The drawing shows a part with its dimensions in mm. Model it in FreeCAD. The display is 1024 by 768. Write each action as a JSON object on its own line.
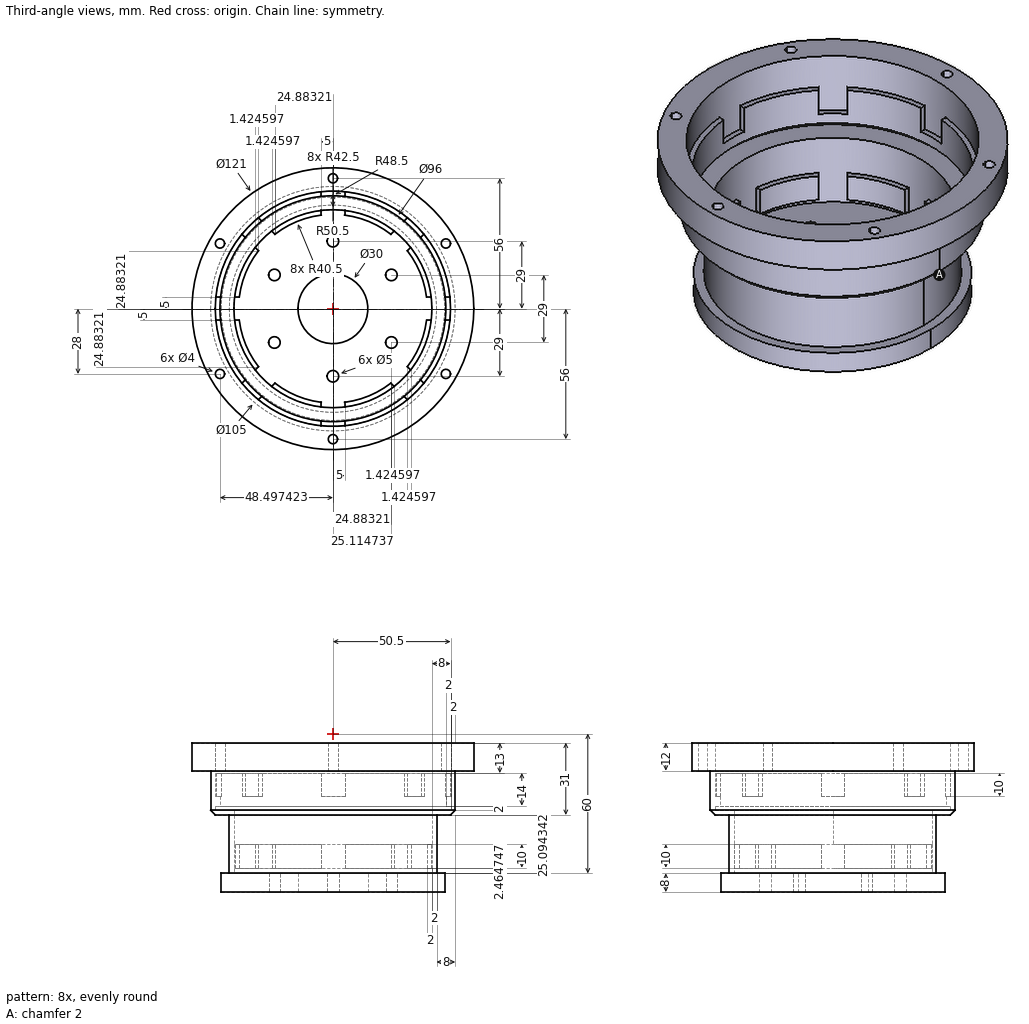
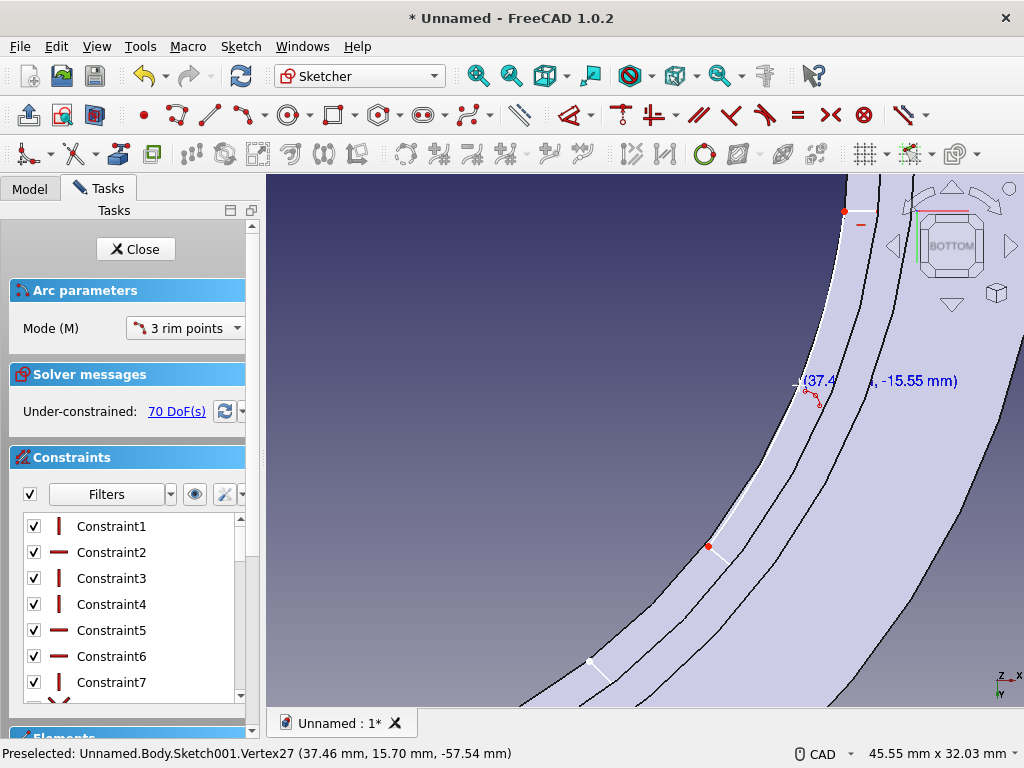
{"action": "left_click", "coordinate": [732, 567]}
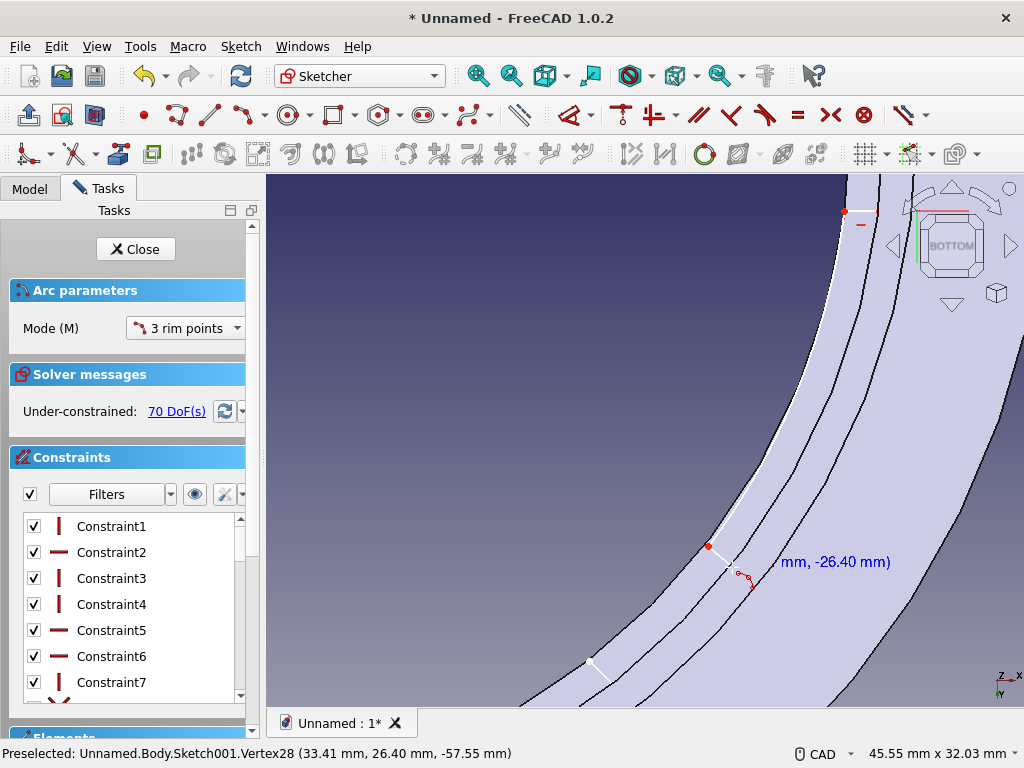
{"action": "scroll", "coordinate": [708, 543], "scroll_direction": "down", "scroll_amount": 7}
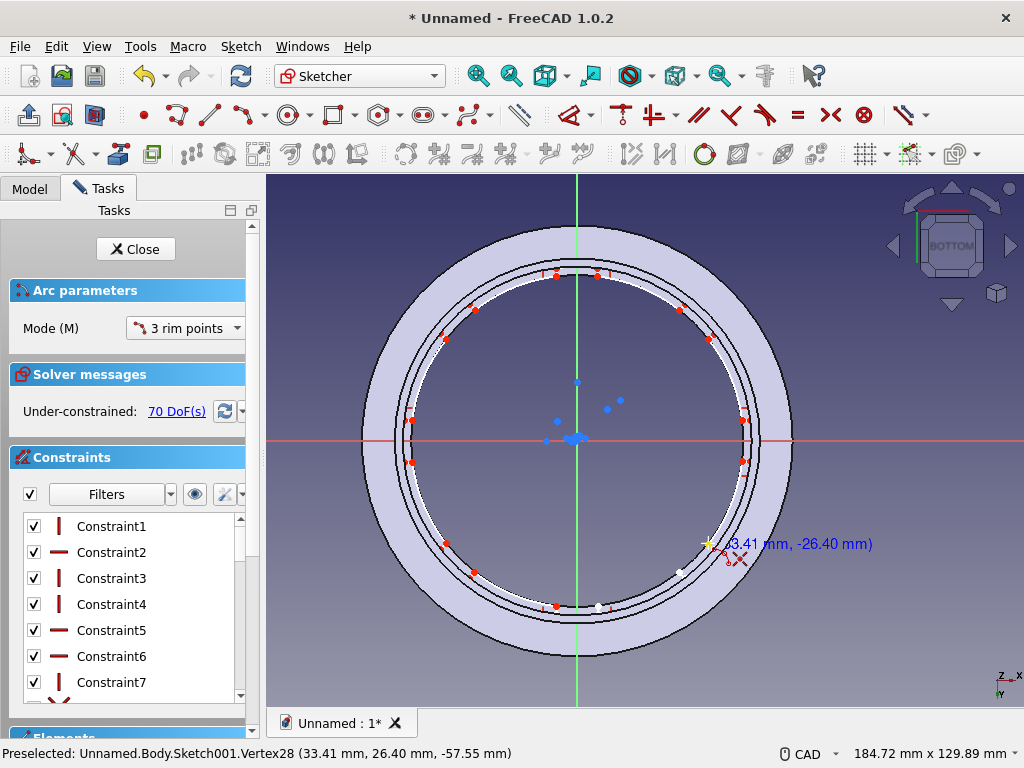
{"action": "scroll", "coordinate": [685, 578], "scroll_direction": "up", "scroll_amount": 7}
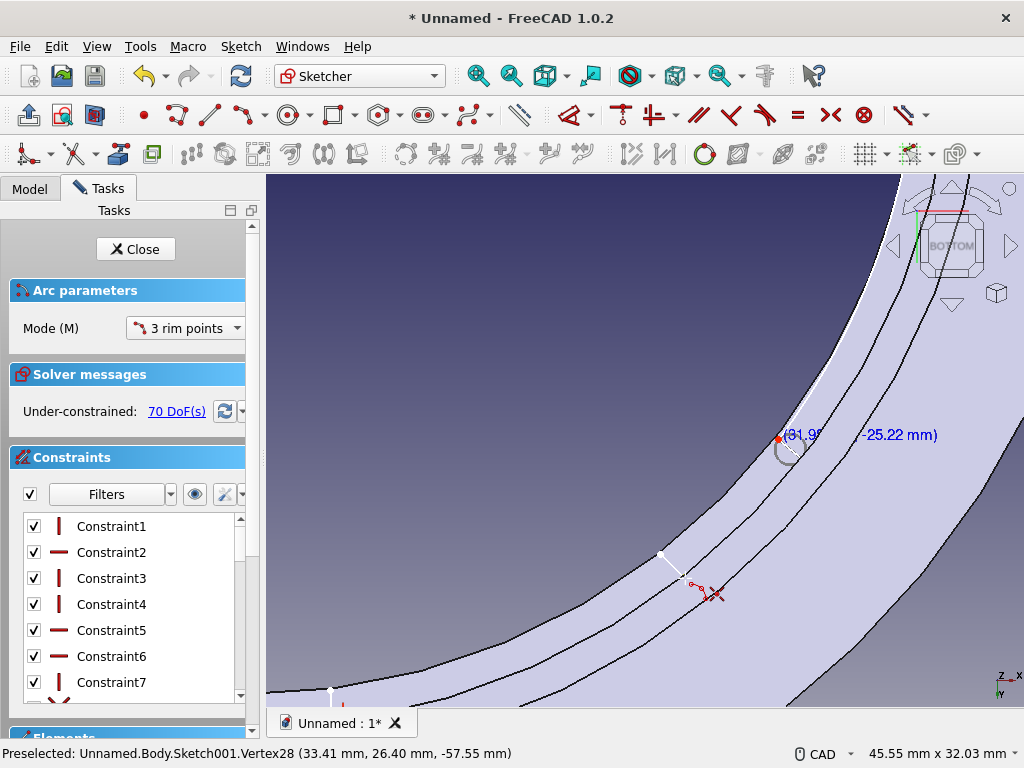
{"action": "left_click", "coordinate": [684, 578]}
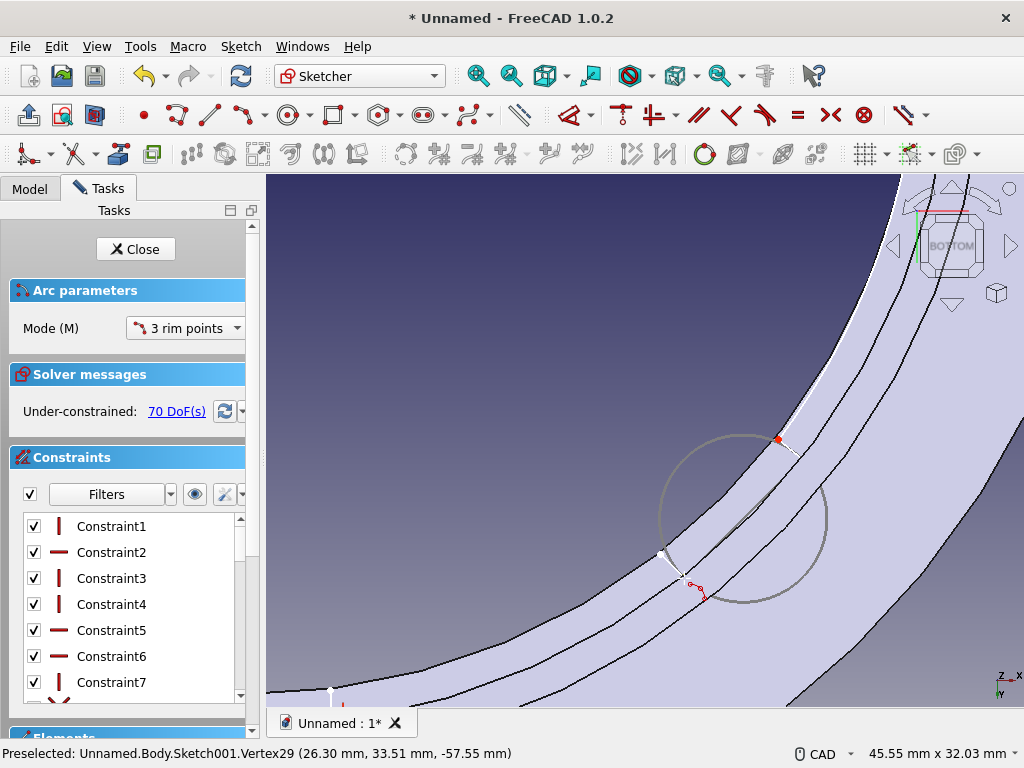
{"action": "scroll", "coordinate": [747, 520], "scroll_direction": "up", "scroll_amount": 6}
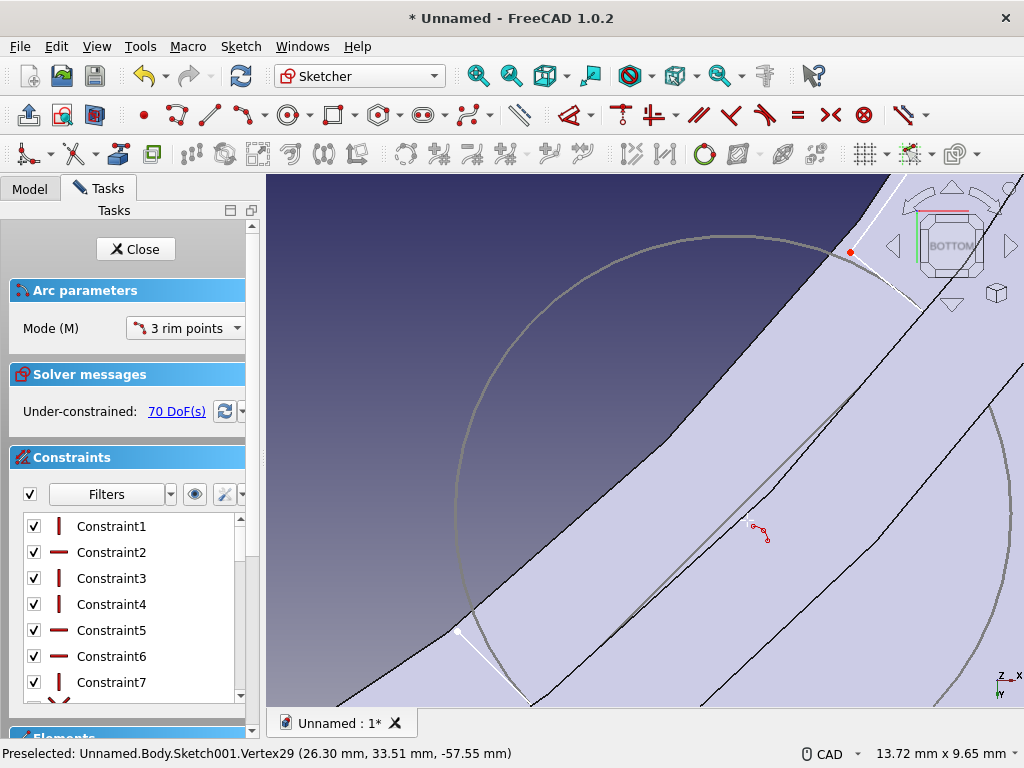
{"action": "left_click", "coordinate": [744, 519]}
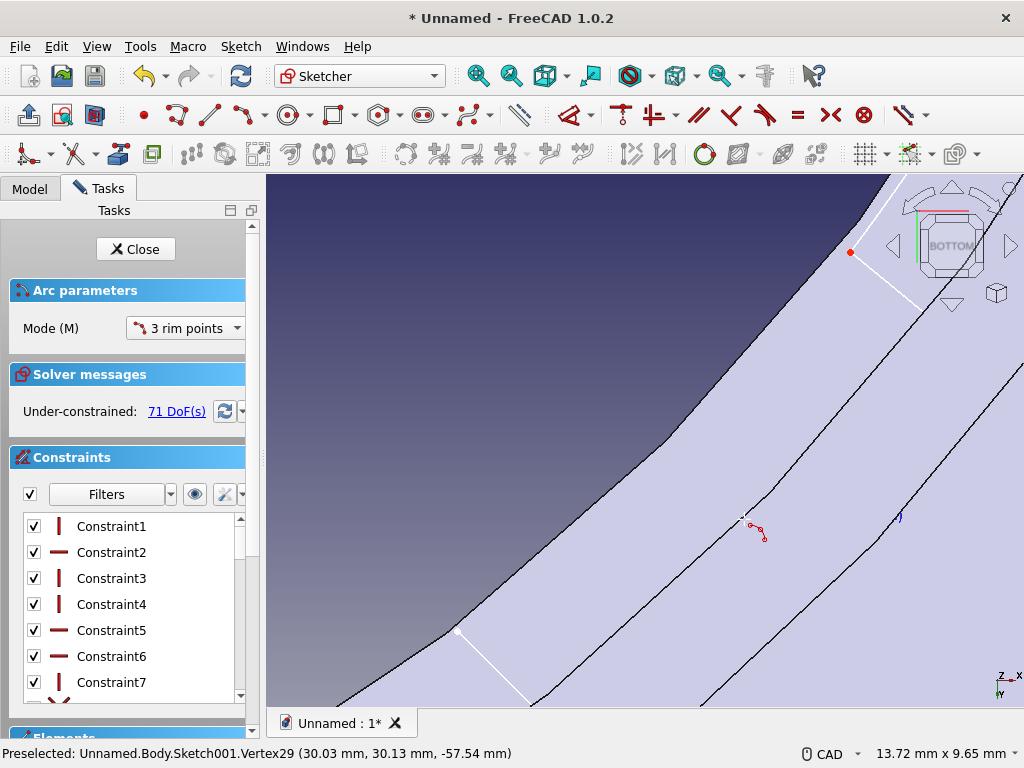
{"action": "scroll", "coordinate": [696, 567], "scroll_direction": "down", "scroll_amount": 13}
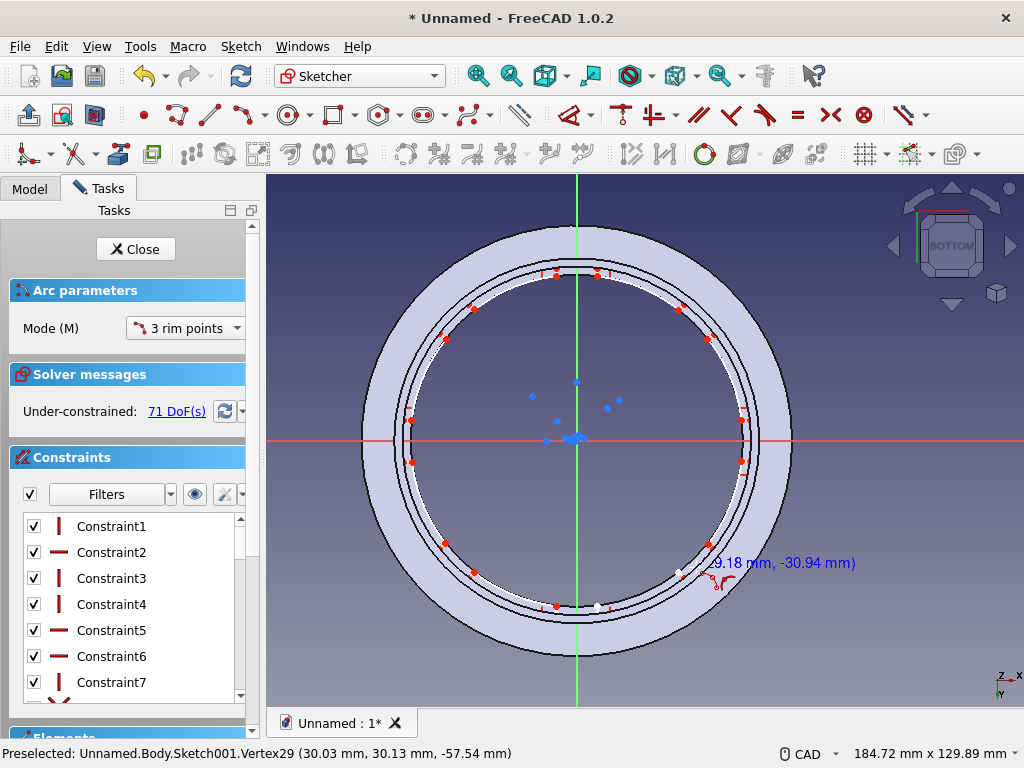
{"action": "scroll", "coordinate": [679, 572], "scroll_direction": "up", "scroll_amount": 7}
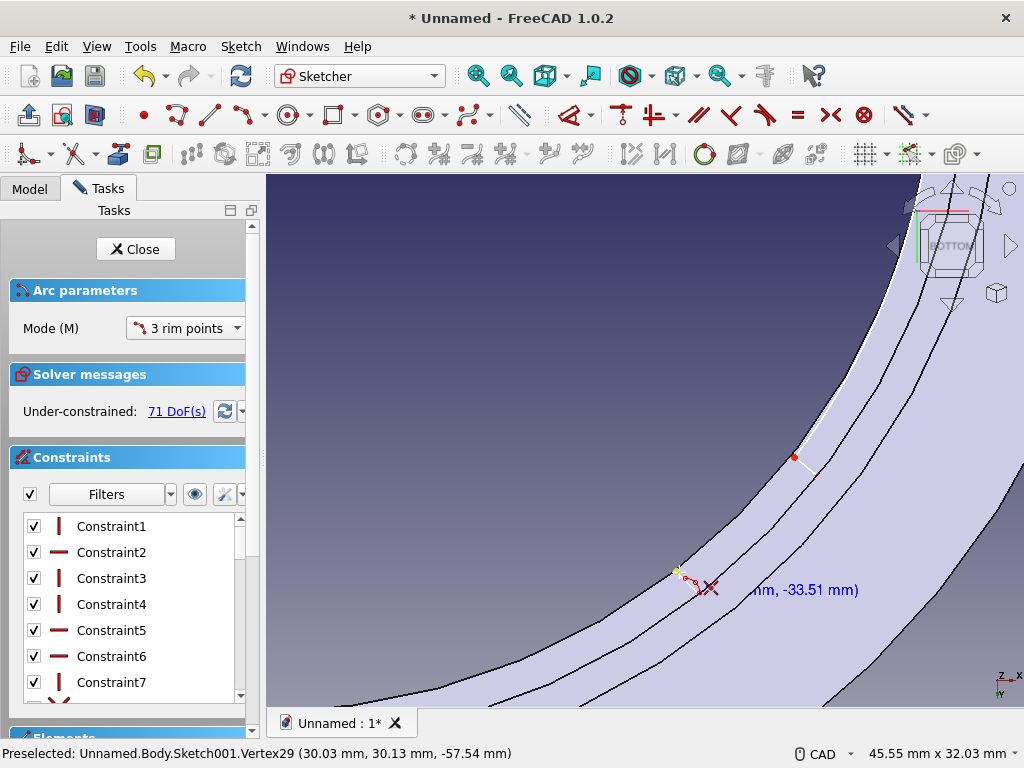
{"action": "left_click", "coordinate": [677, 572]}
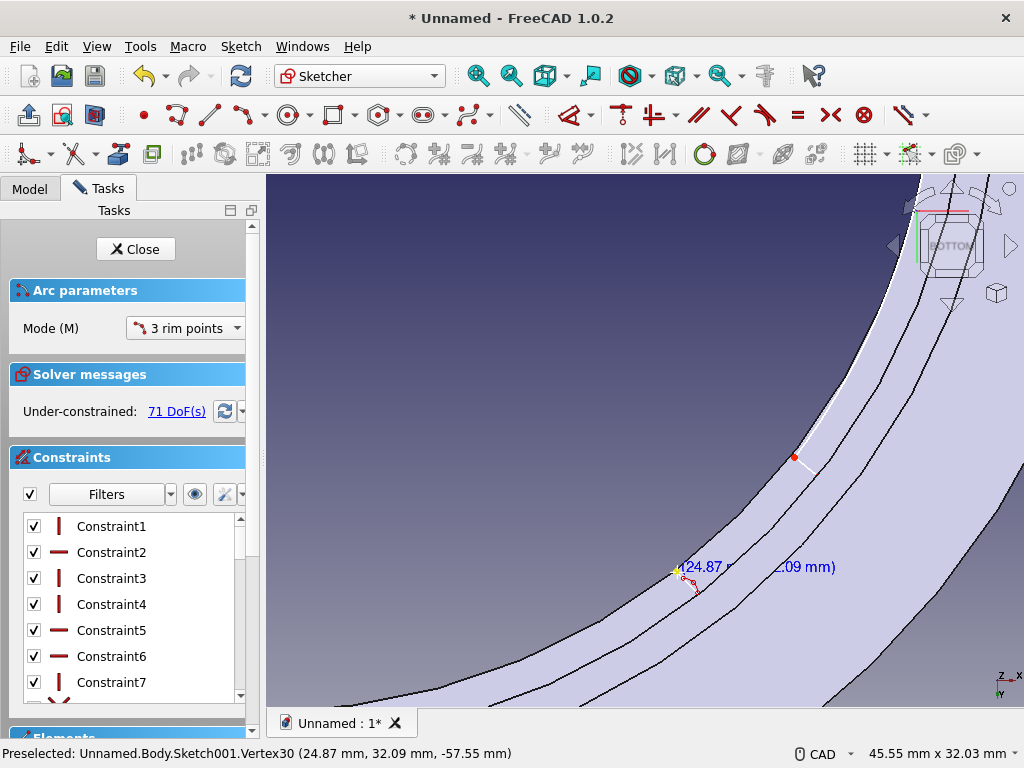
{"action": "scroll", "coordinate": [679, 572], "scroll_direction": "down", "scroll_amount": 7}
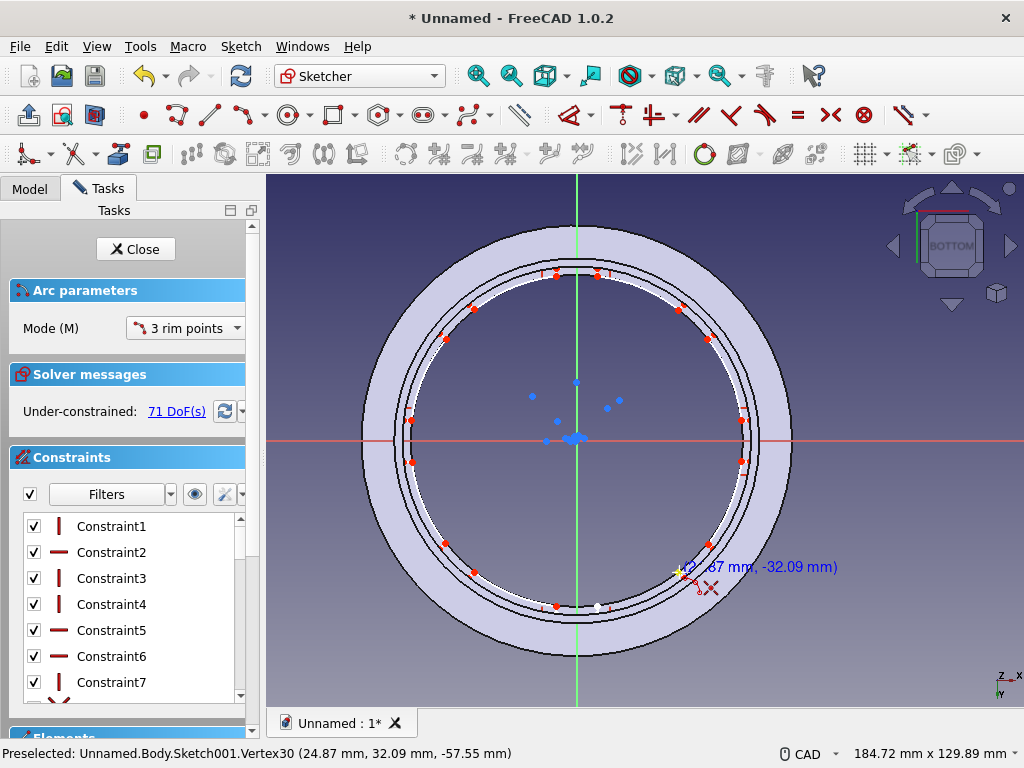
{"action": "scroll", "coordinate": [597, 606], "scroll_direction": "up", "scroll_amount": 7}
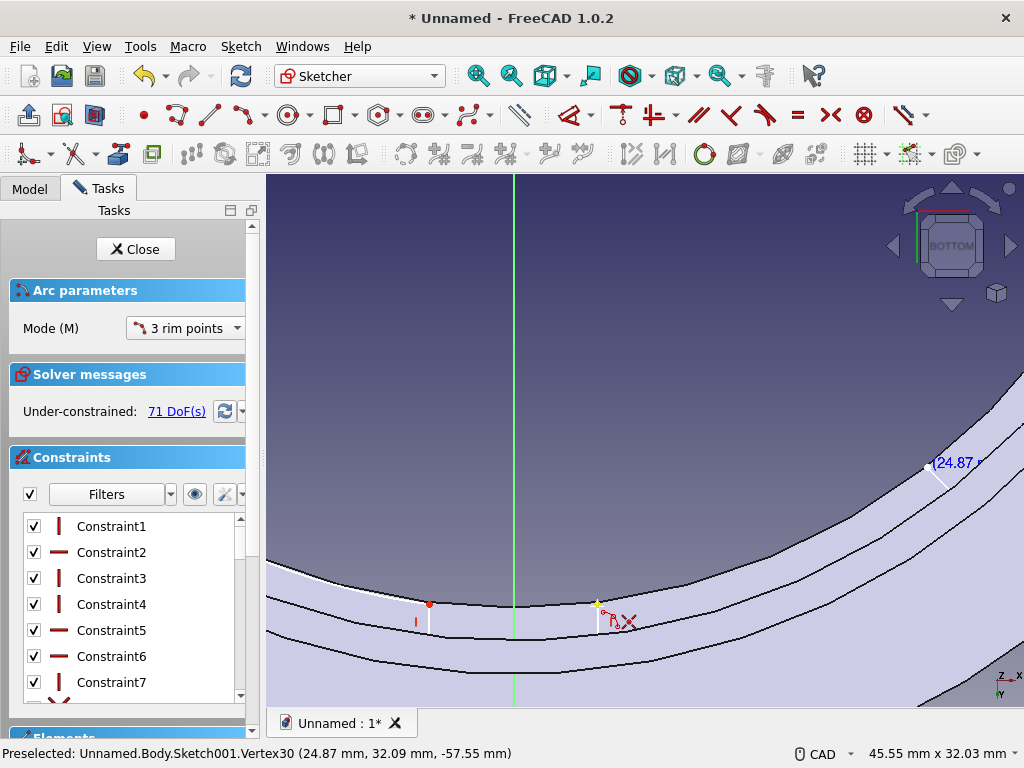
{"action": "left_click", "coordinate": [598, 604]}
{"action": "left_click", "coordinate": [772, 556]}